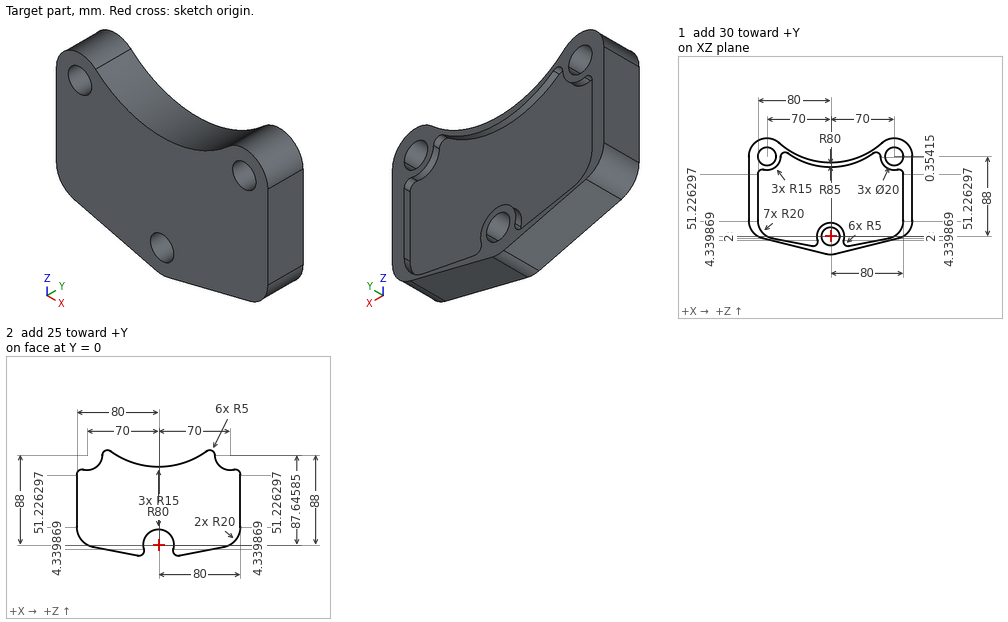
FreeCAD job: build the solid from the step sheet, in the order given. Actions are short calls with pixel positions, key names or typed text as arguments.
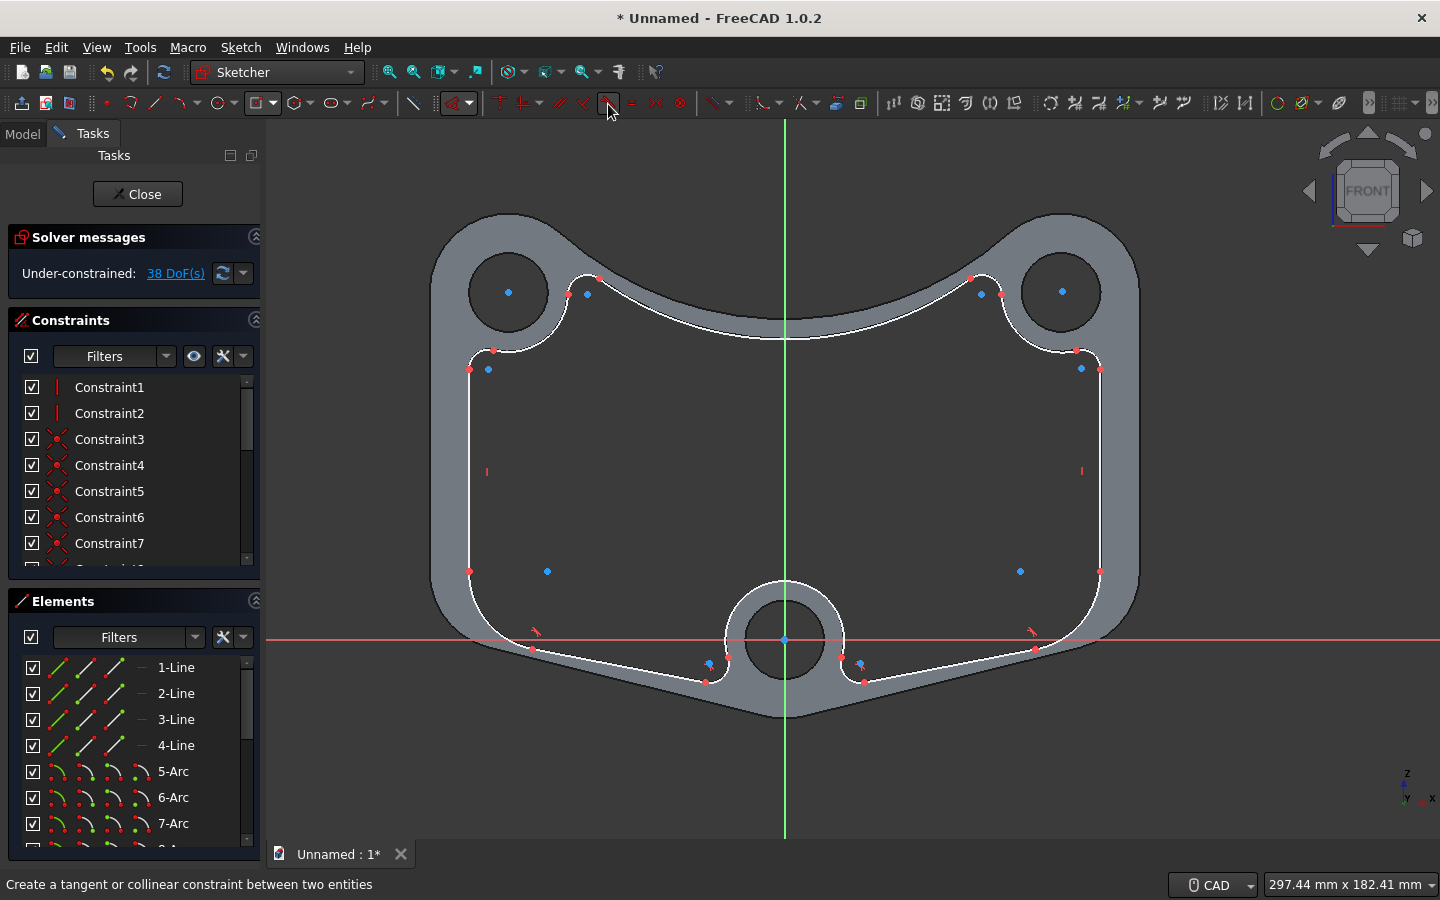
click(1100, 511)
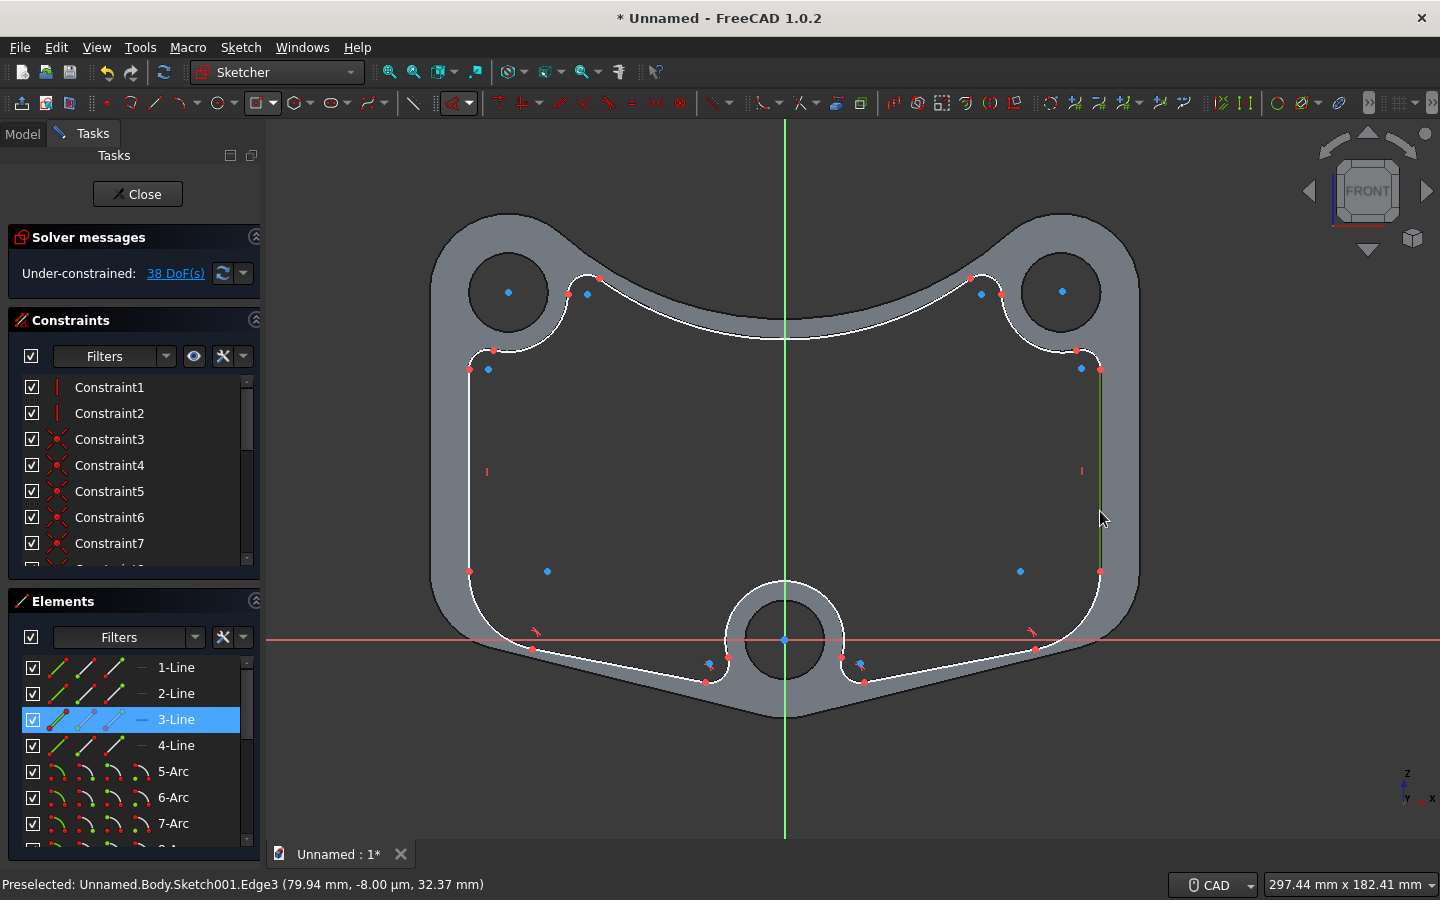
click(1066, 637)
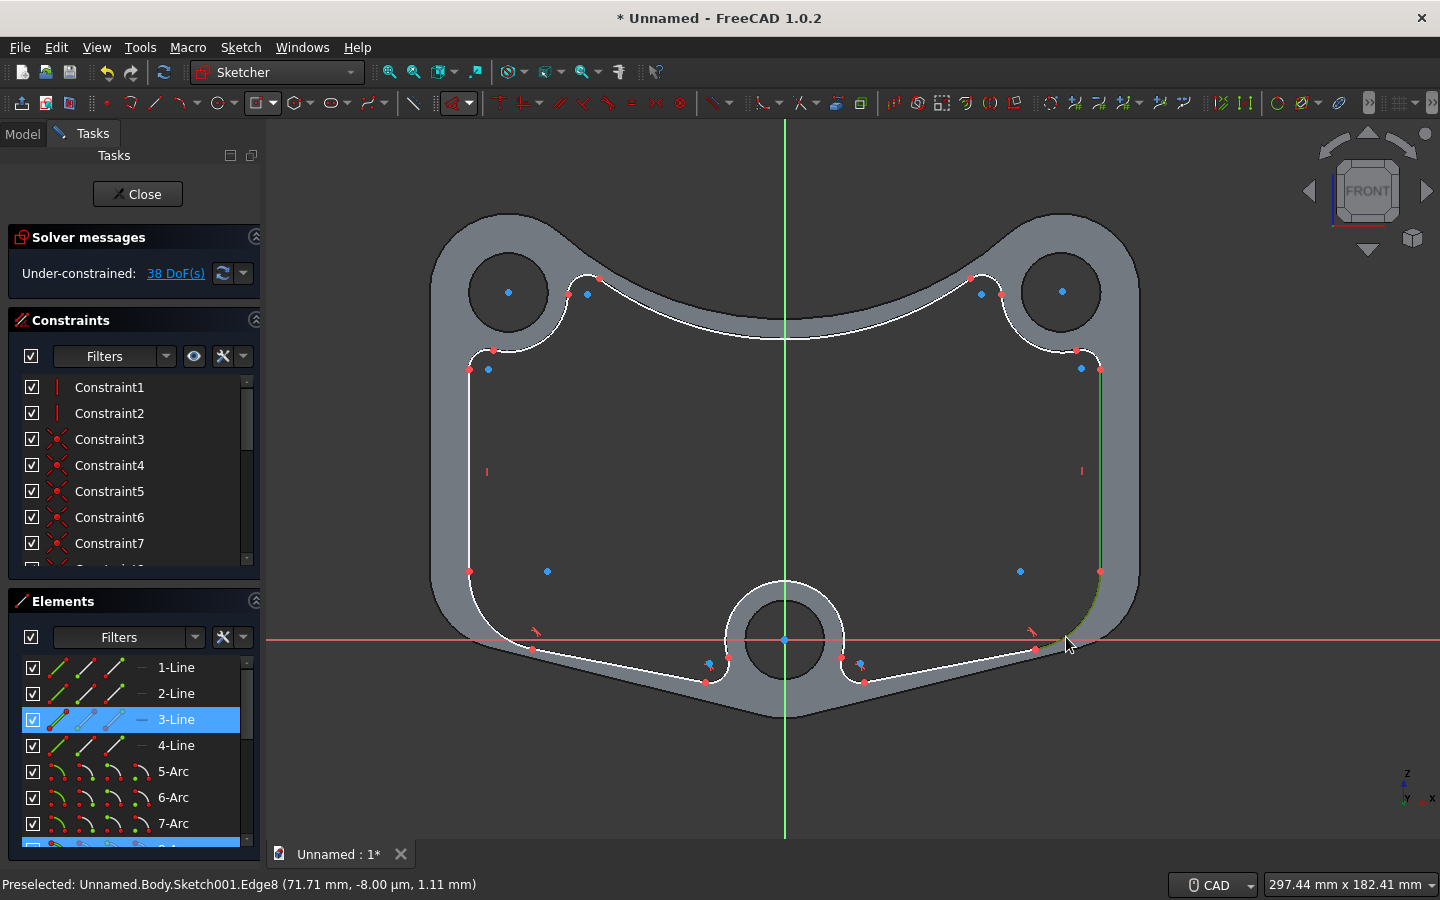
click(608, 104)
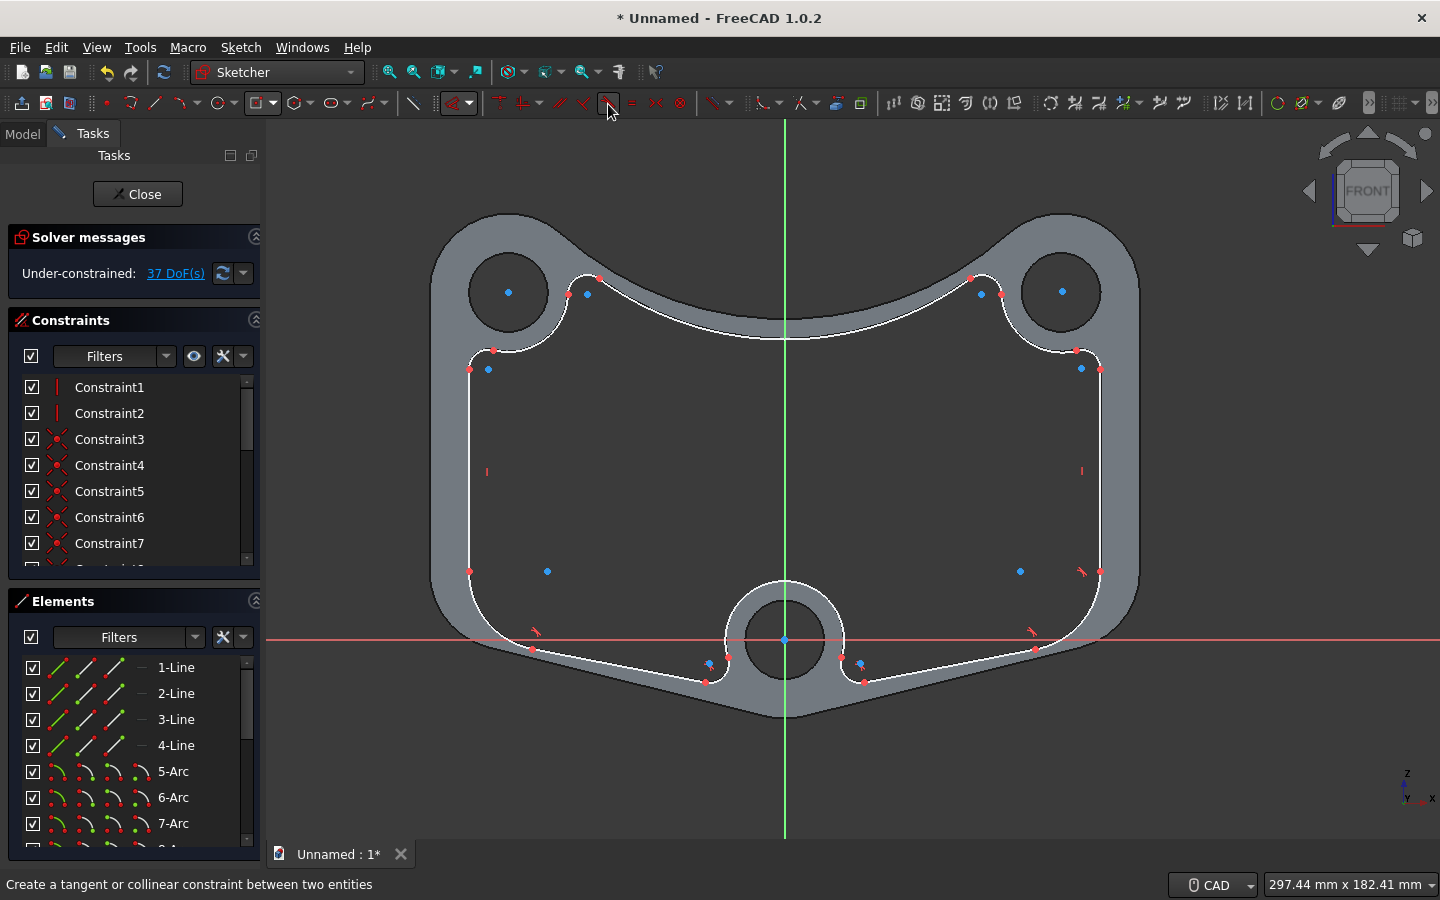
click(1100, 511)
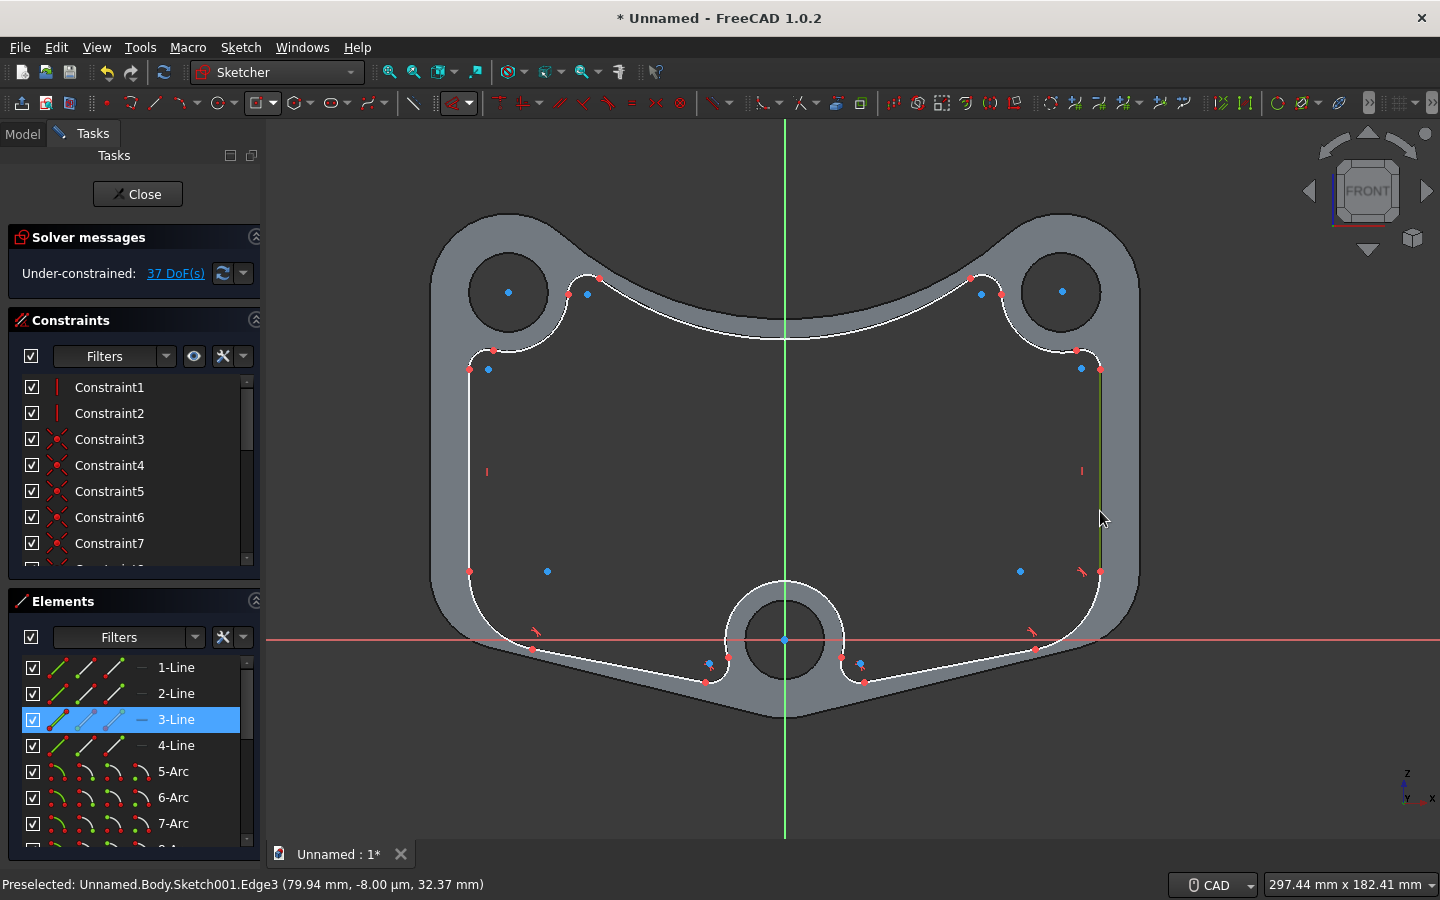
scroll(1098, 359, up, 2)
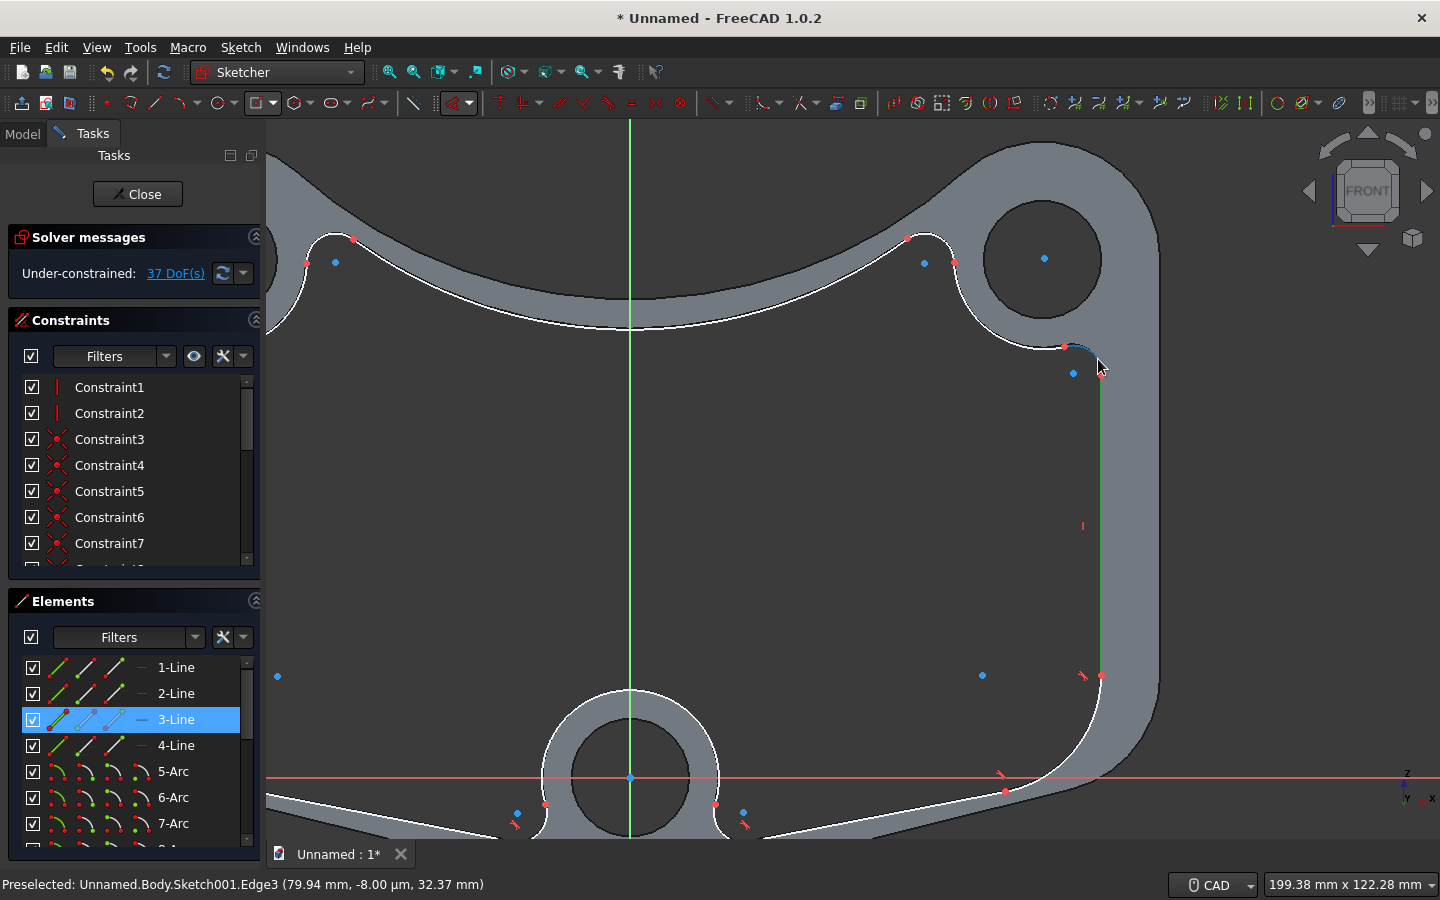
click(1098, 360)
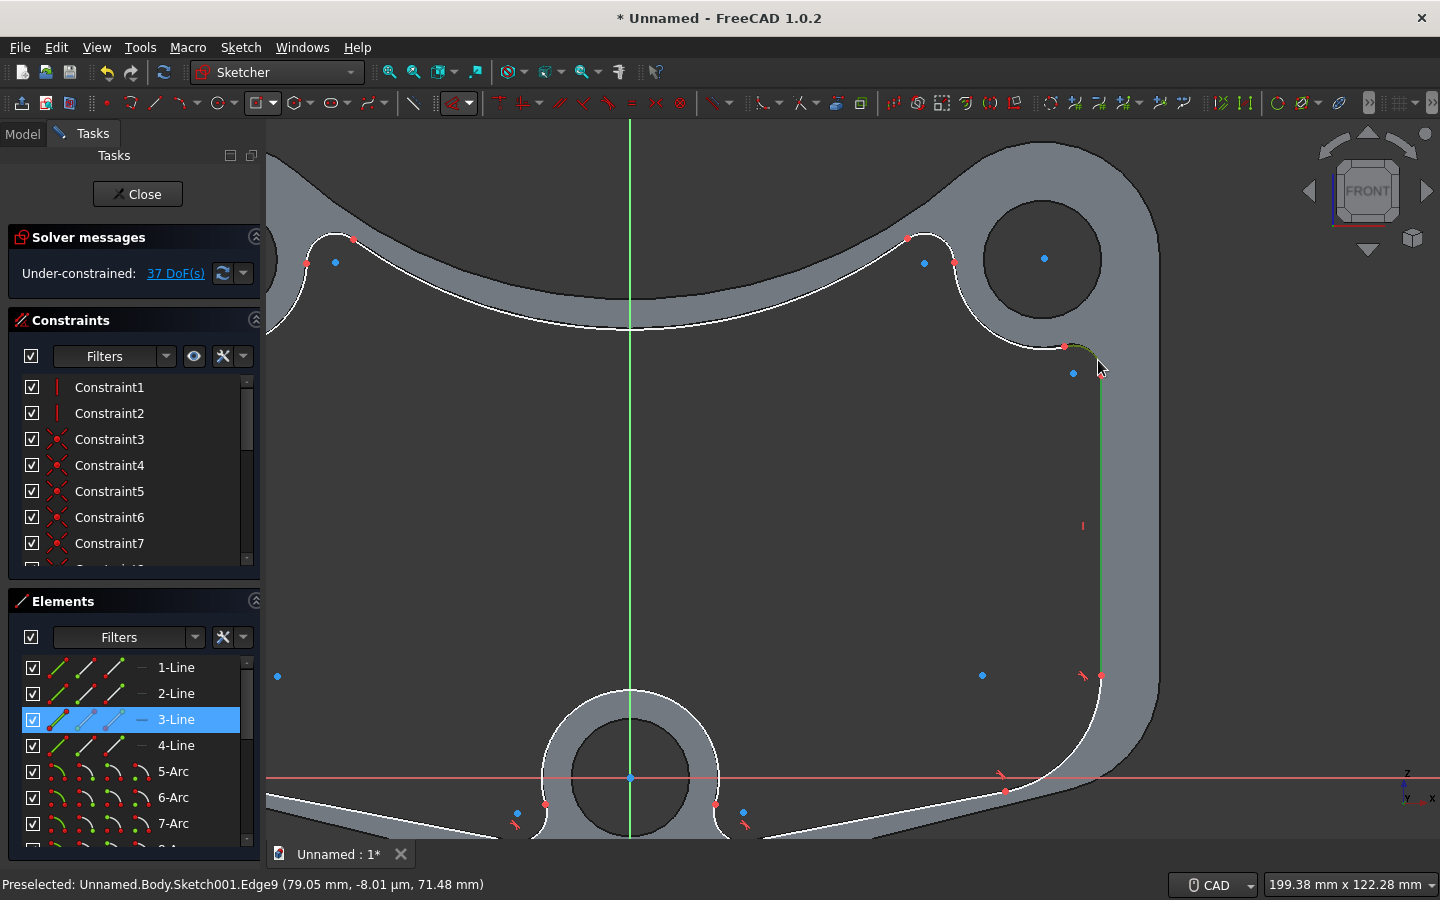
click(608, 104)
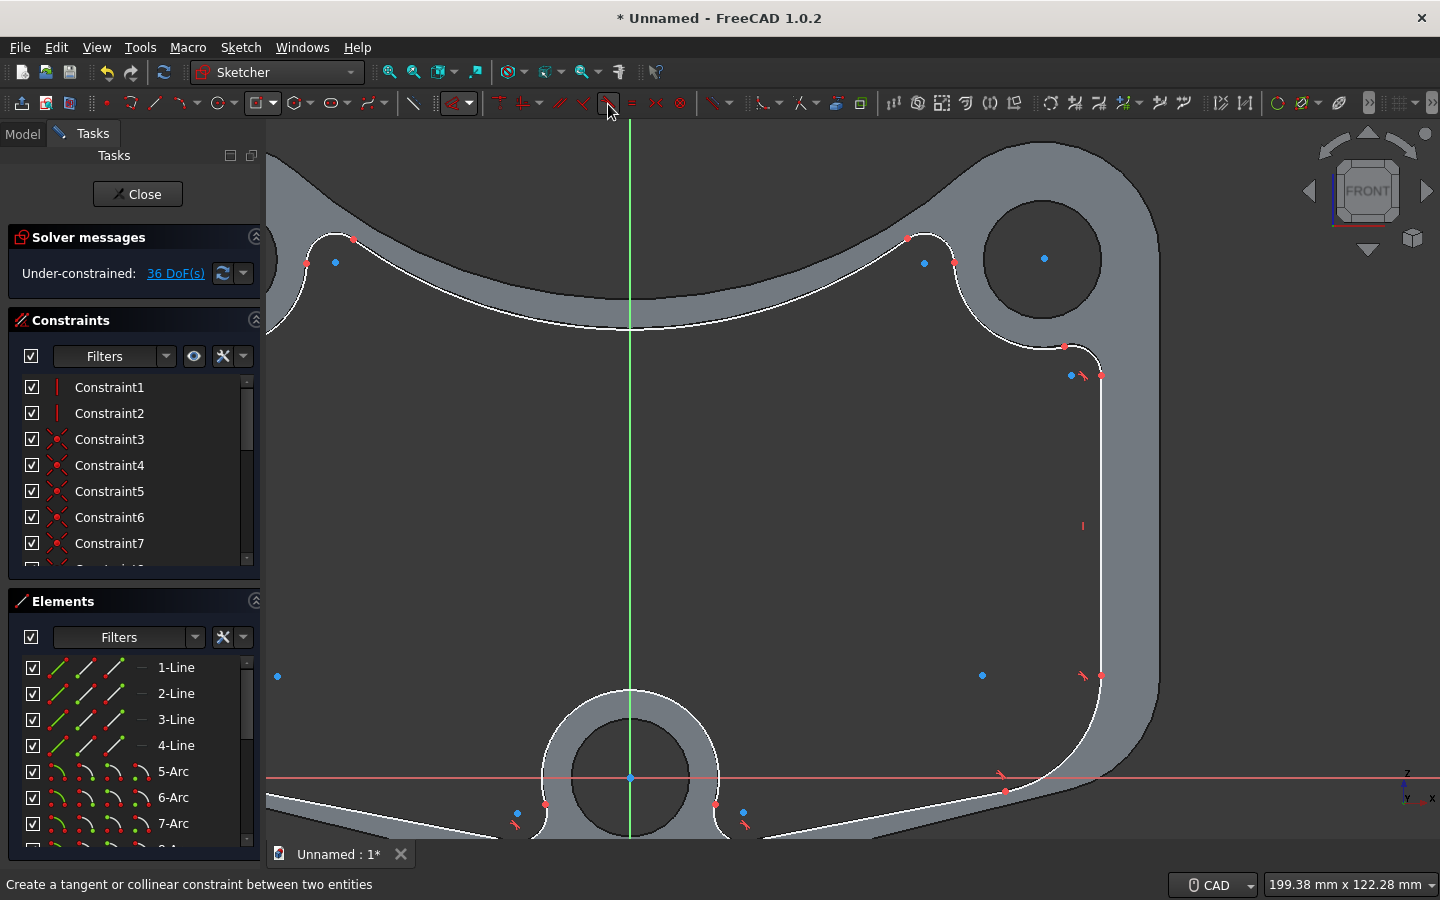
scroll(1098, 358, down, 2)